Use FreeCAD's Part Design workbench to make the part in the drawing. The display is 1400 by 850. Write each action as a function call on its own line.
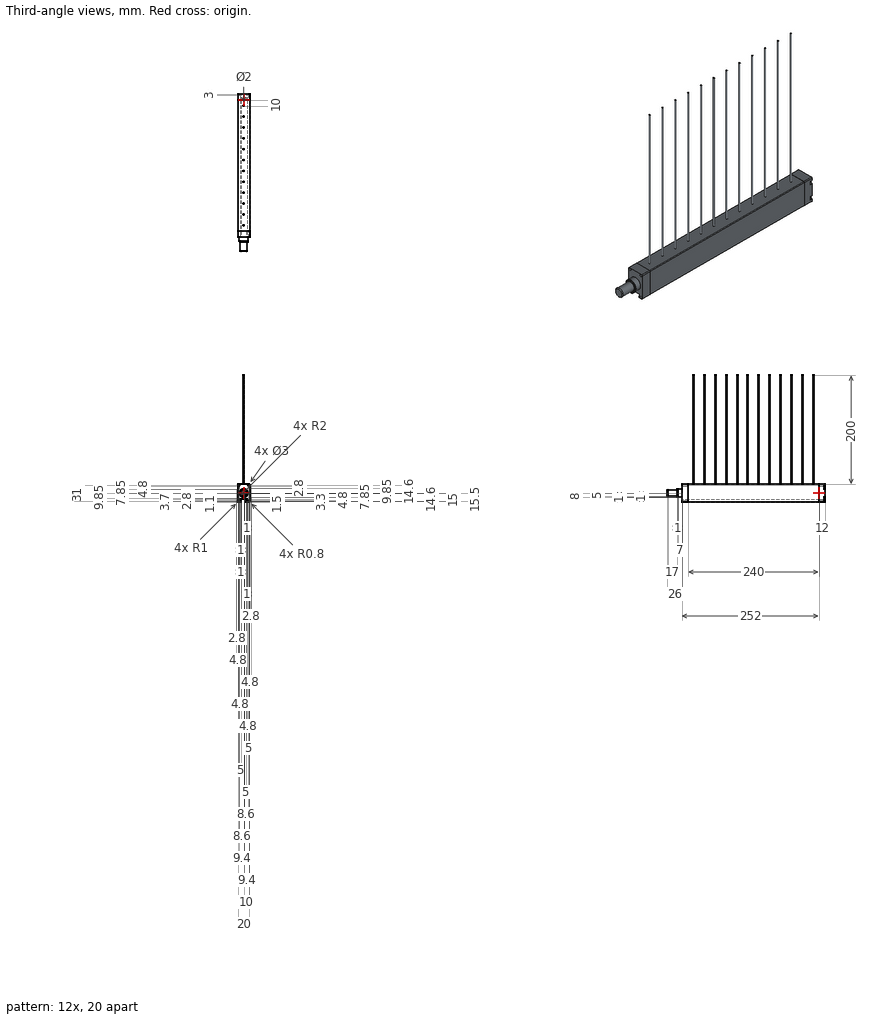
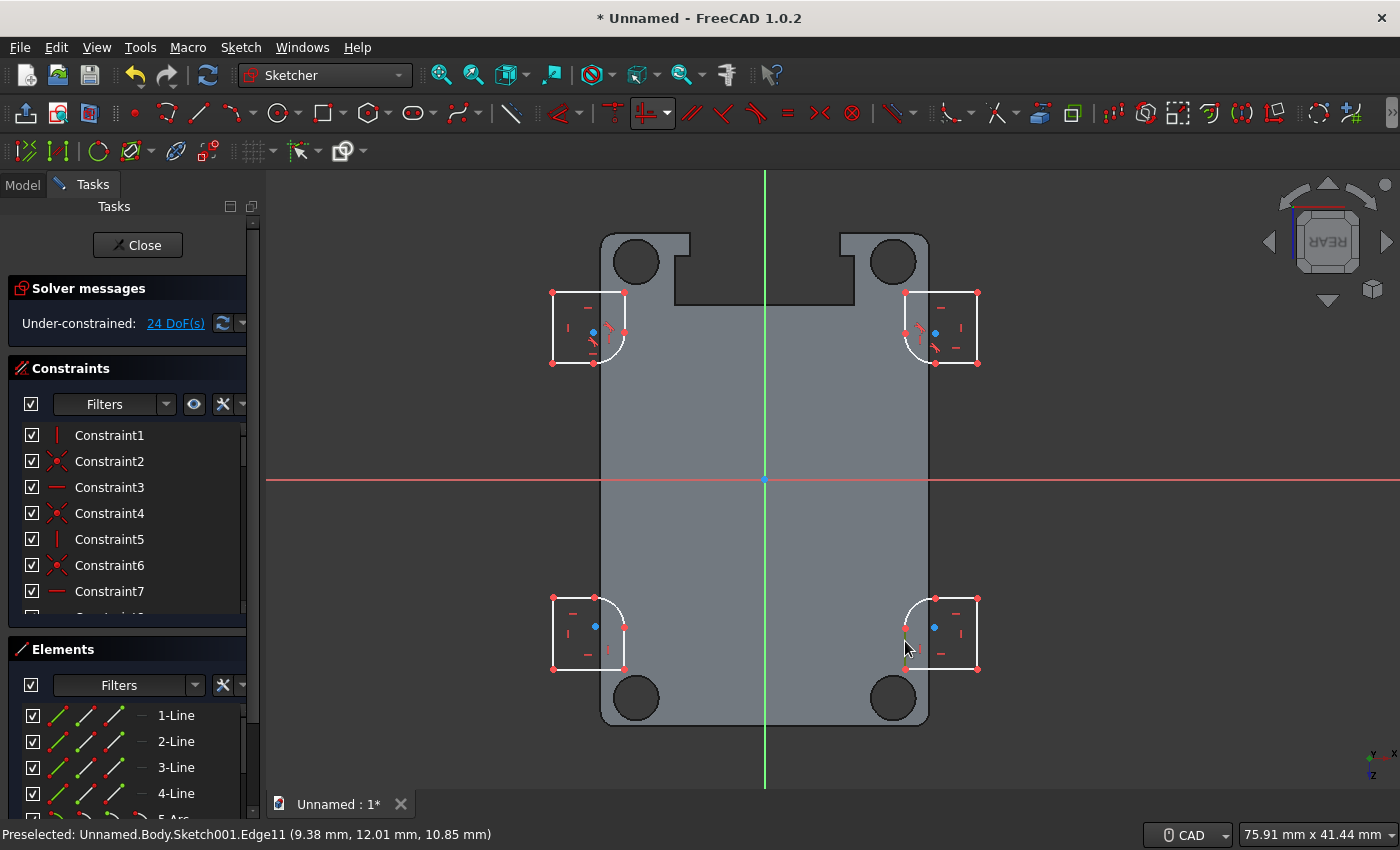
click(921, 601)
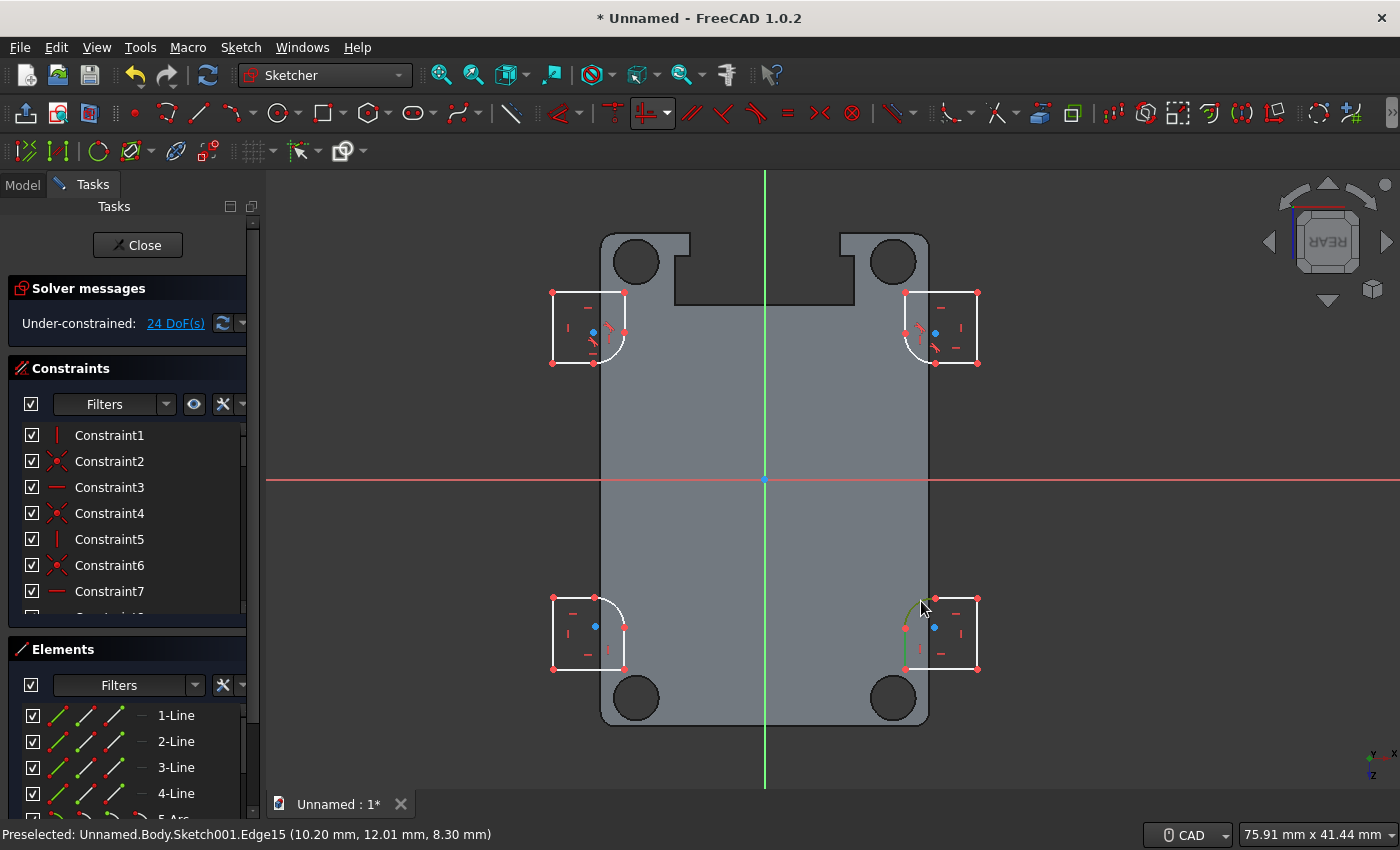
click(756, 114)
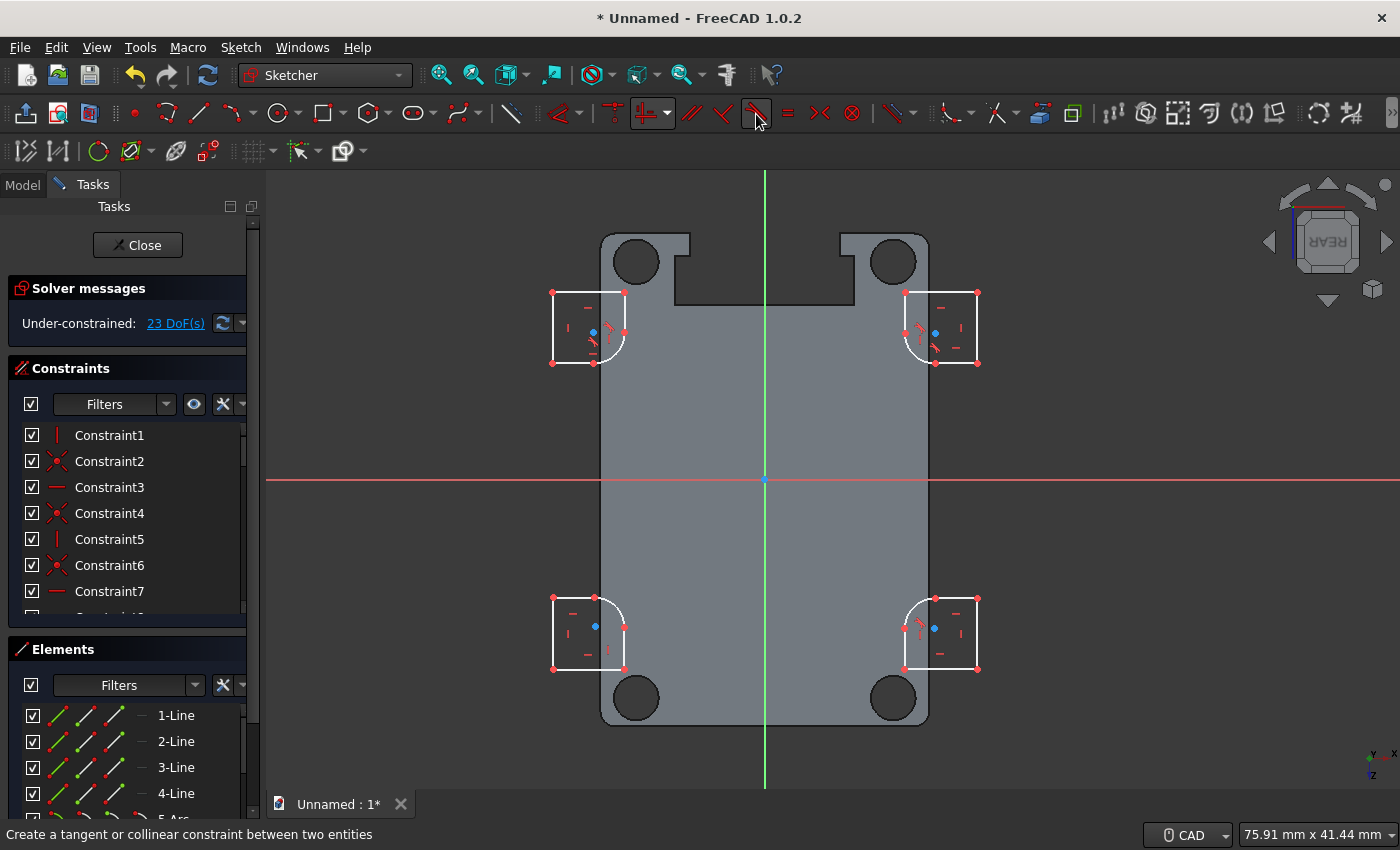
click(964, 598)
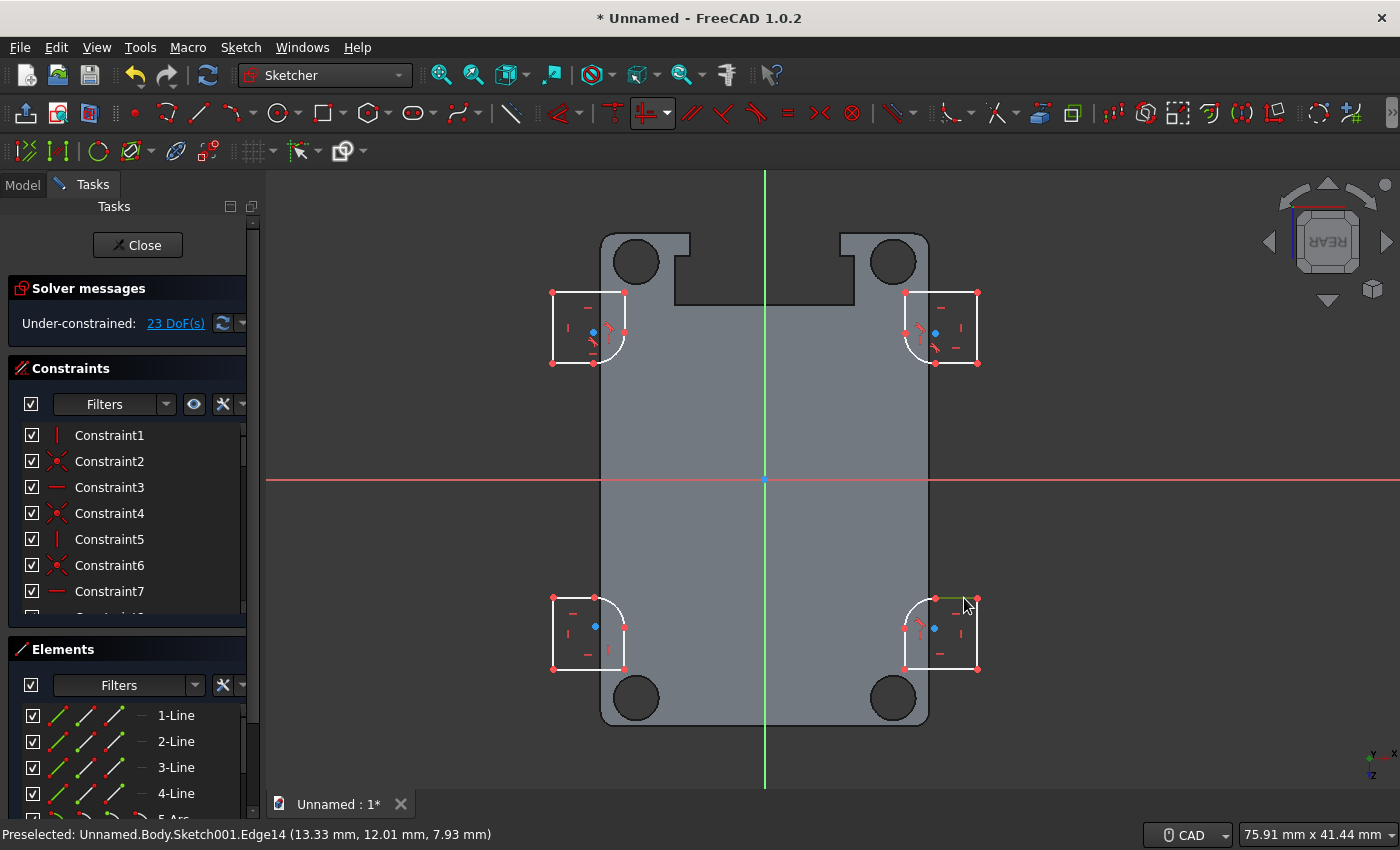
click(921, 602)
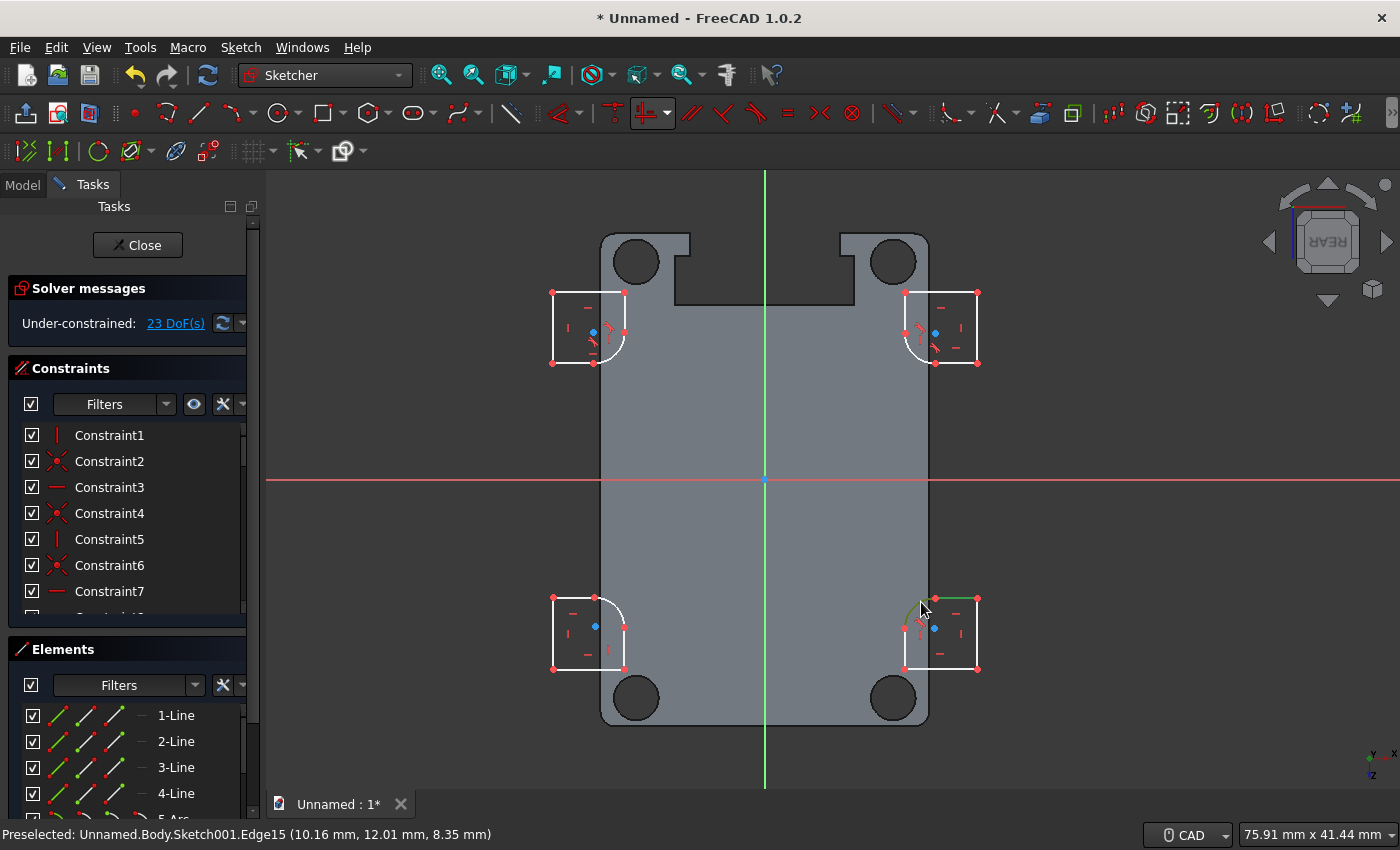
click(756, 114)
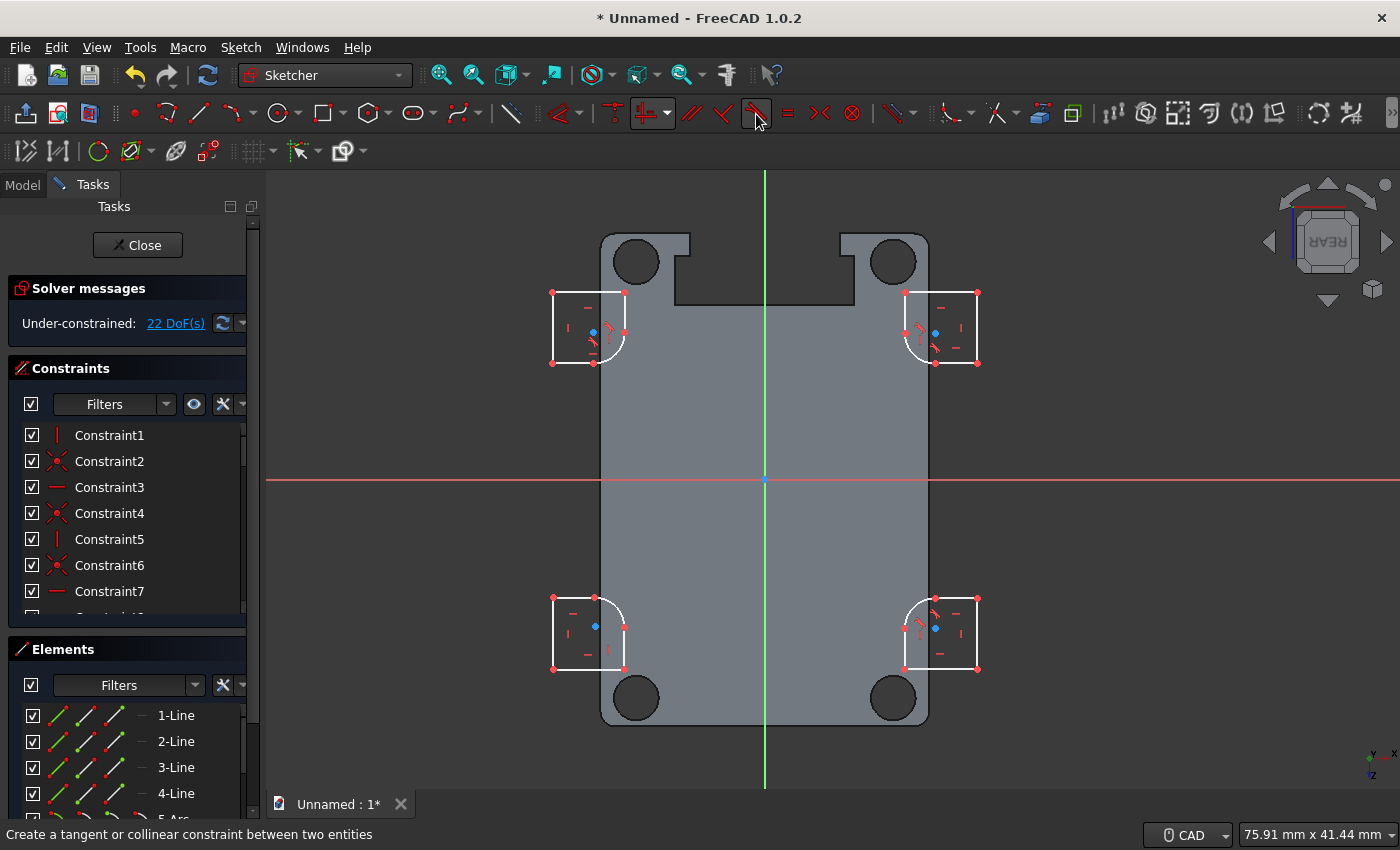
click(582, 598)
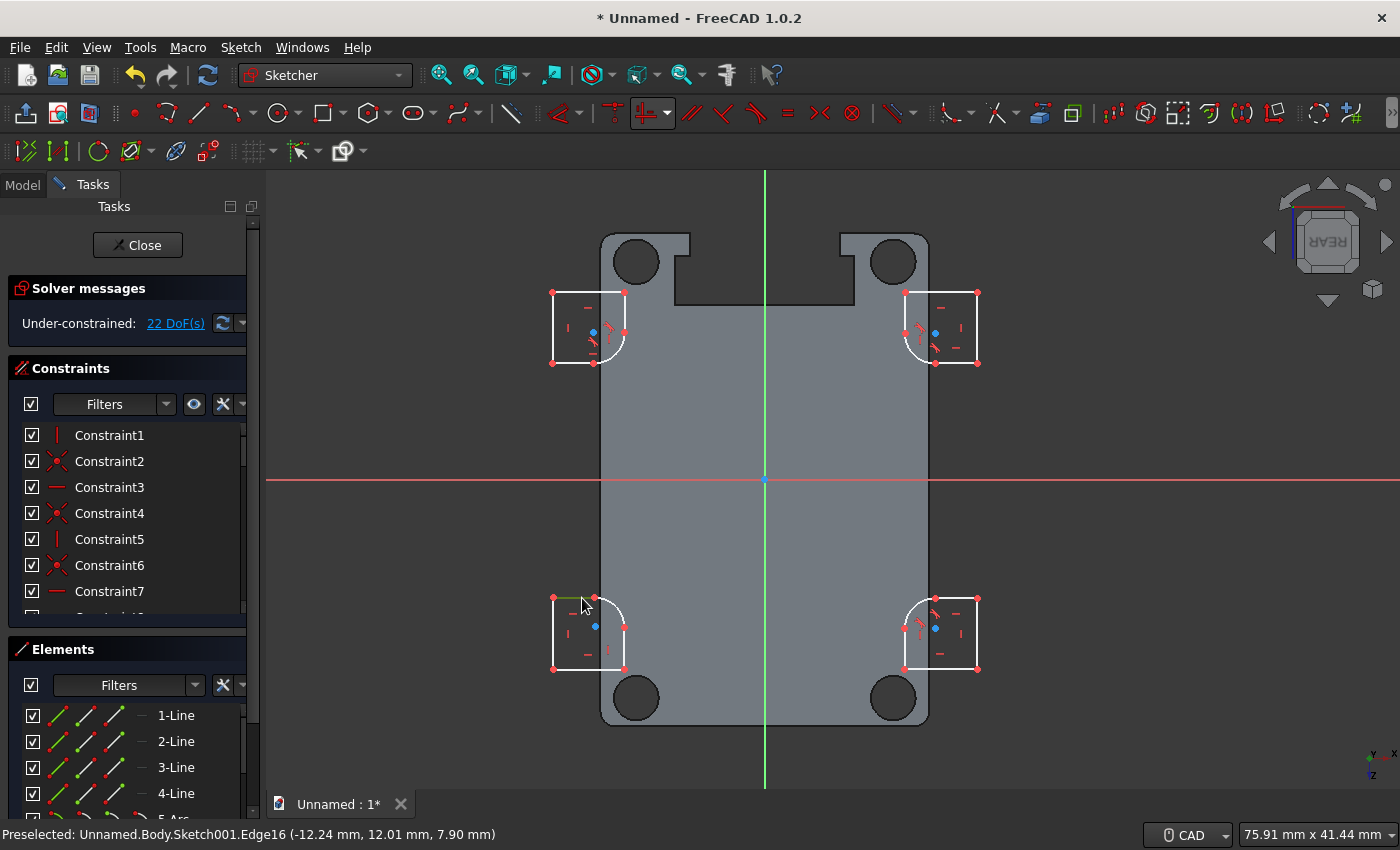
click(621, 614)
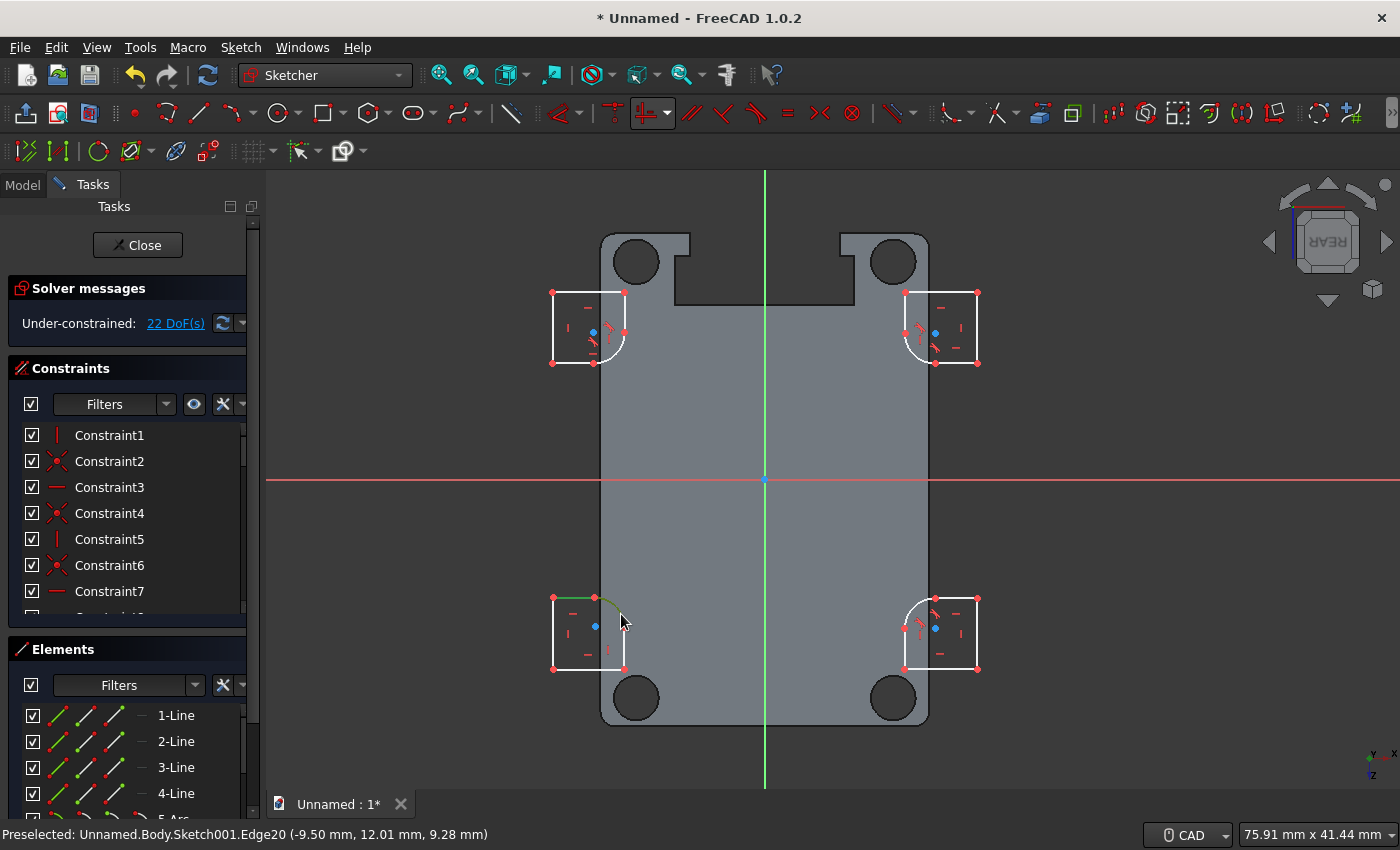
click(756, 114)